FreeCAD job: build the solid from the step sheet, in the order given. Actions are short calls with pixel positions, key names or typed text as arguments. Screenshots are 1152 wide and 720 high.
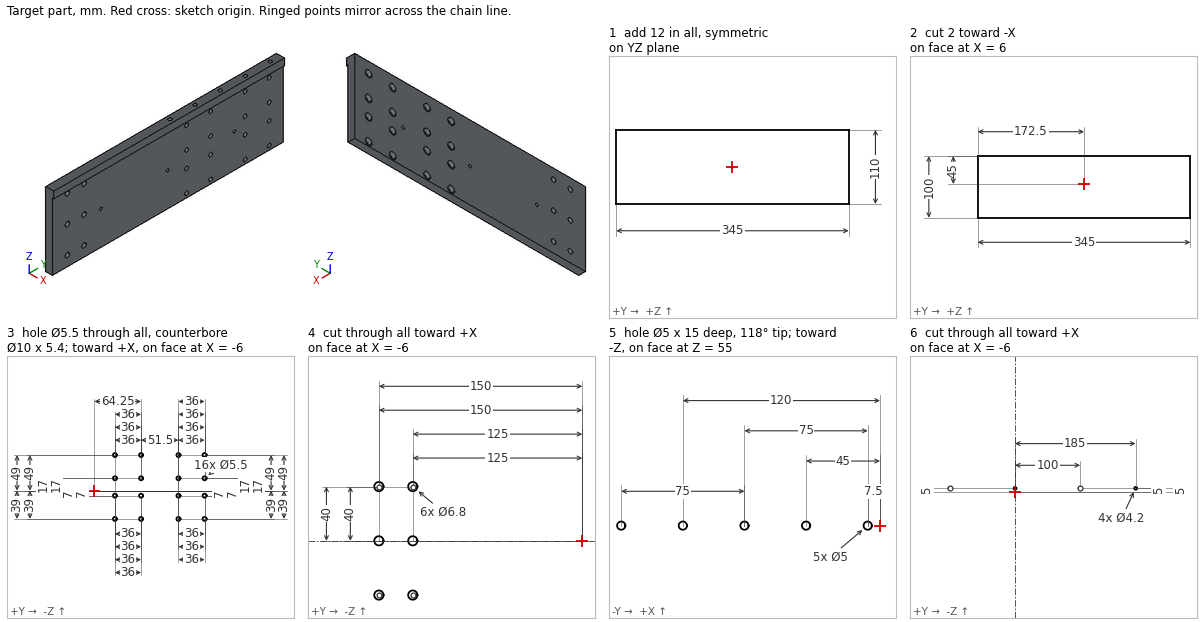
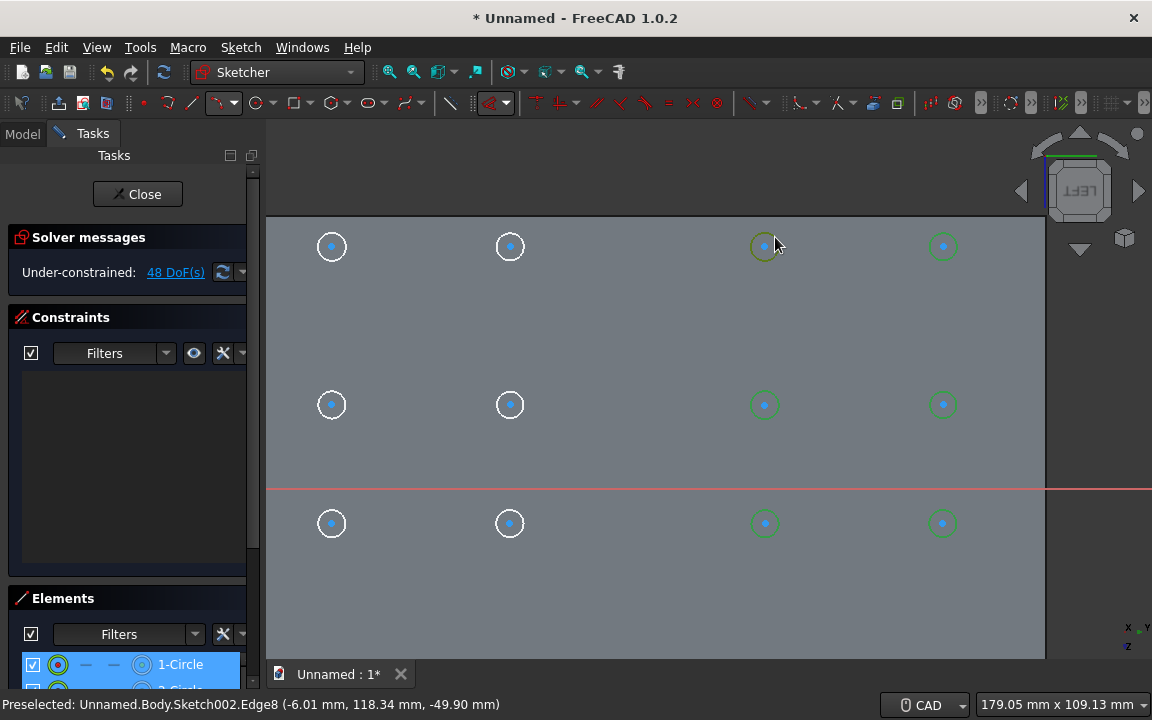
click(520, 237)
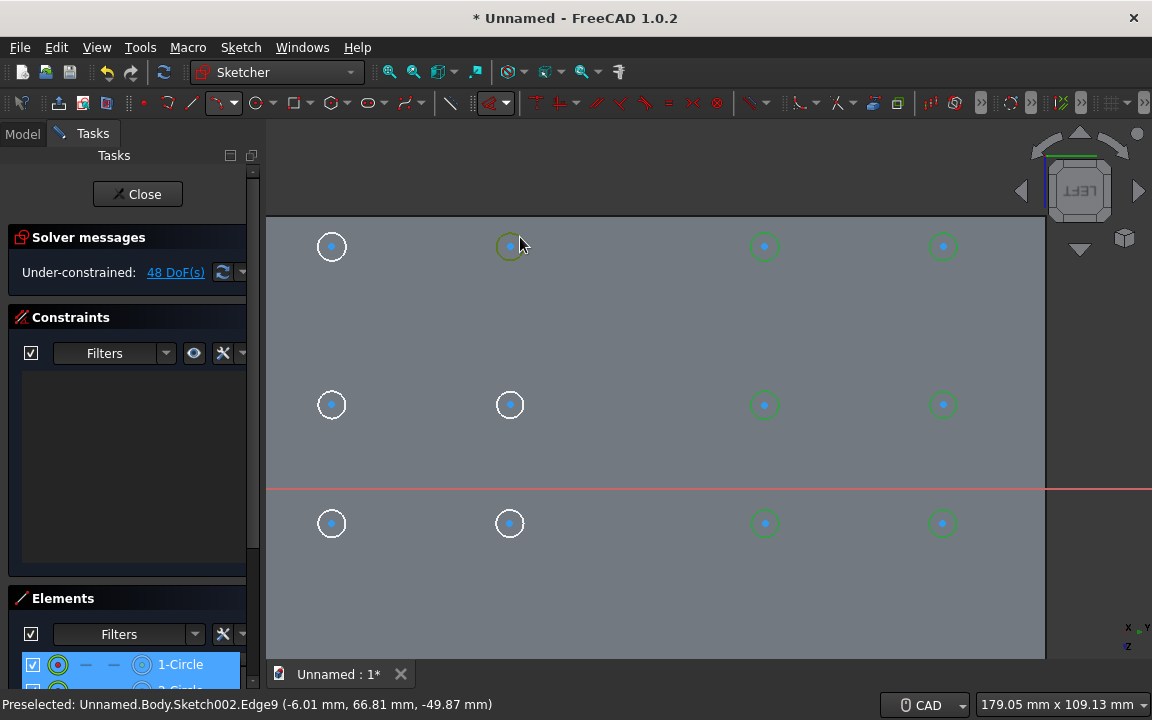
click(342, 237)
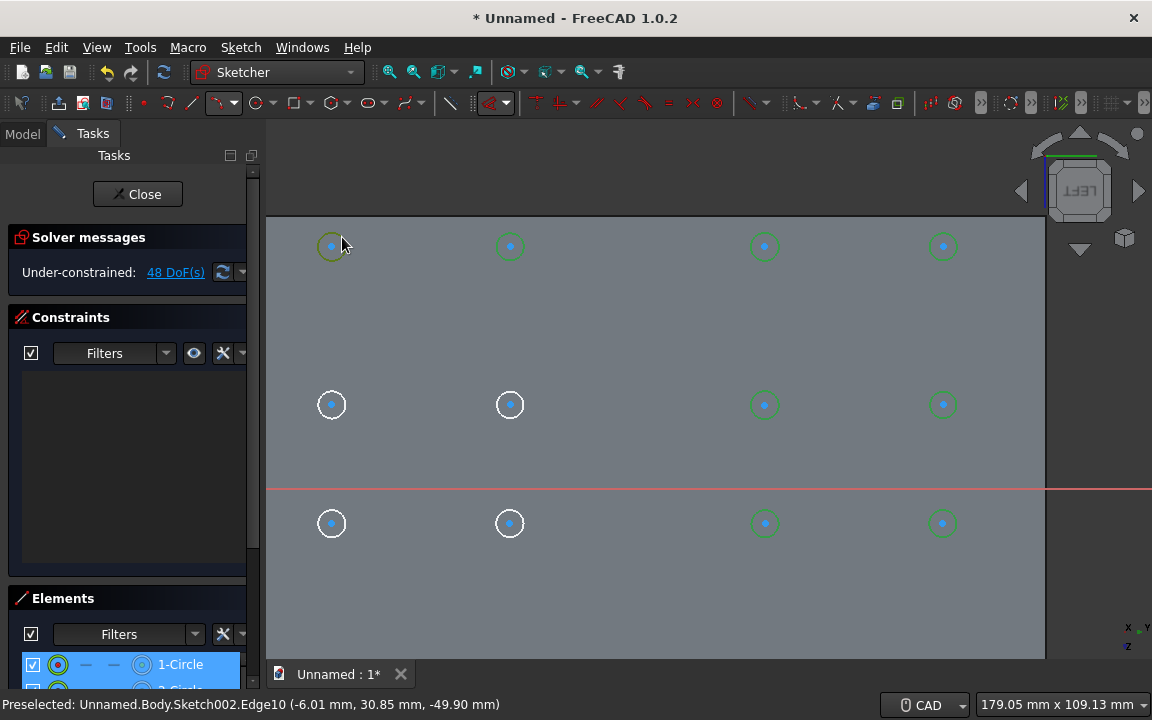
click(520, 396)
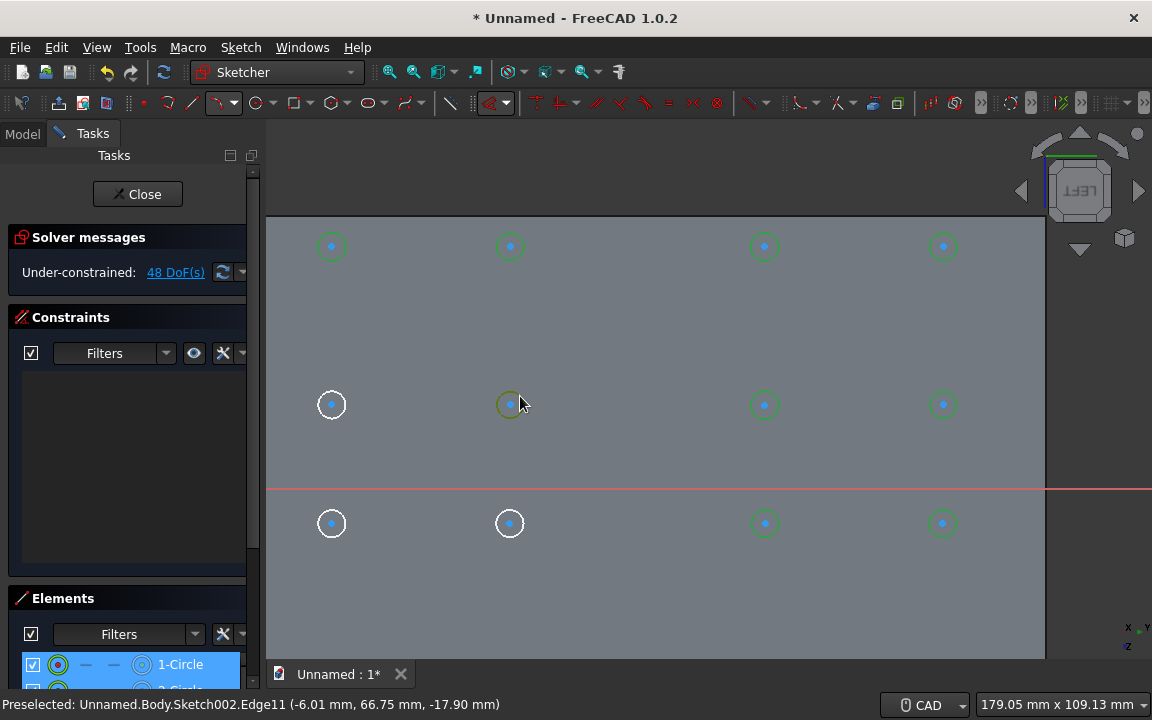
click(341, 395)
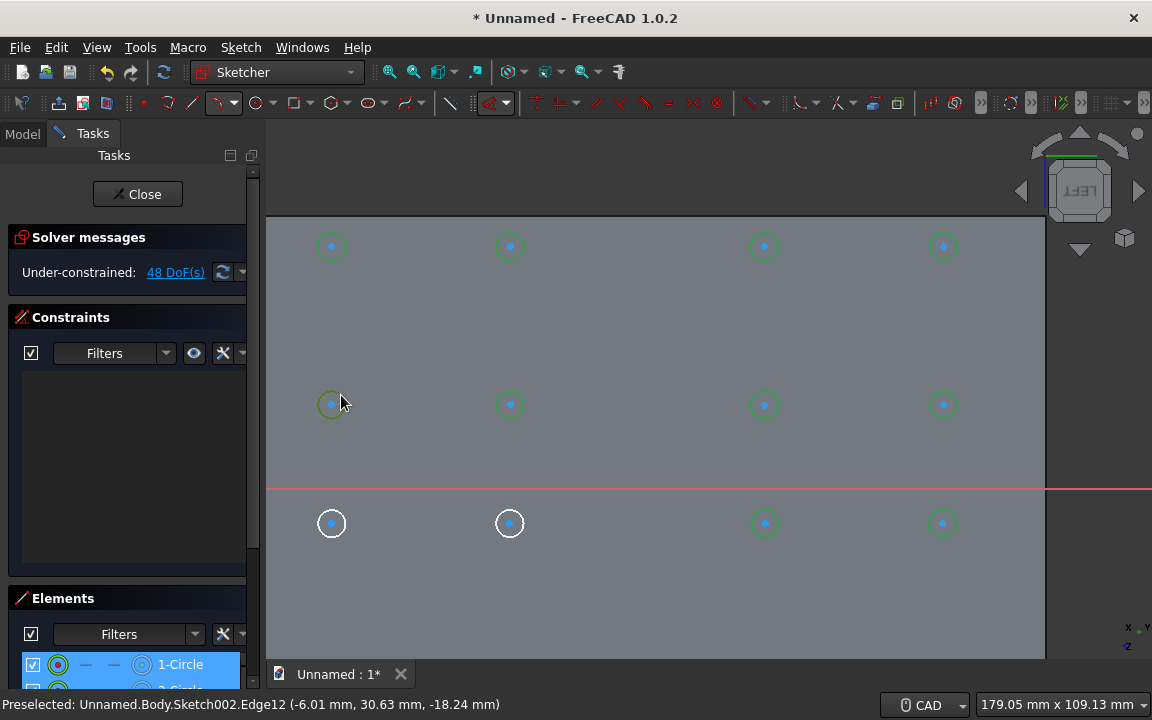
click(519, 514)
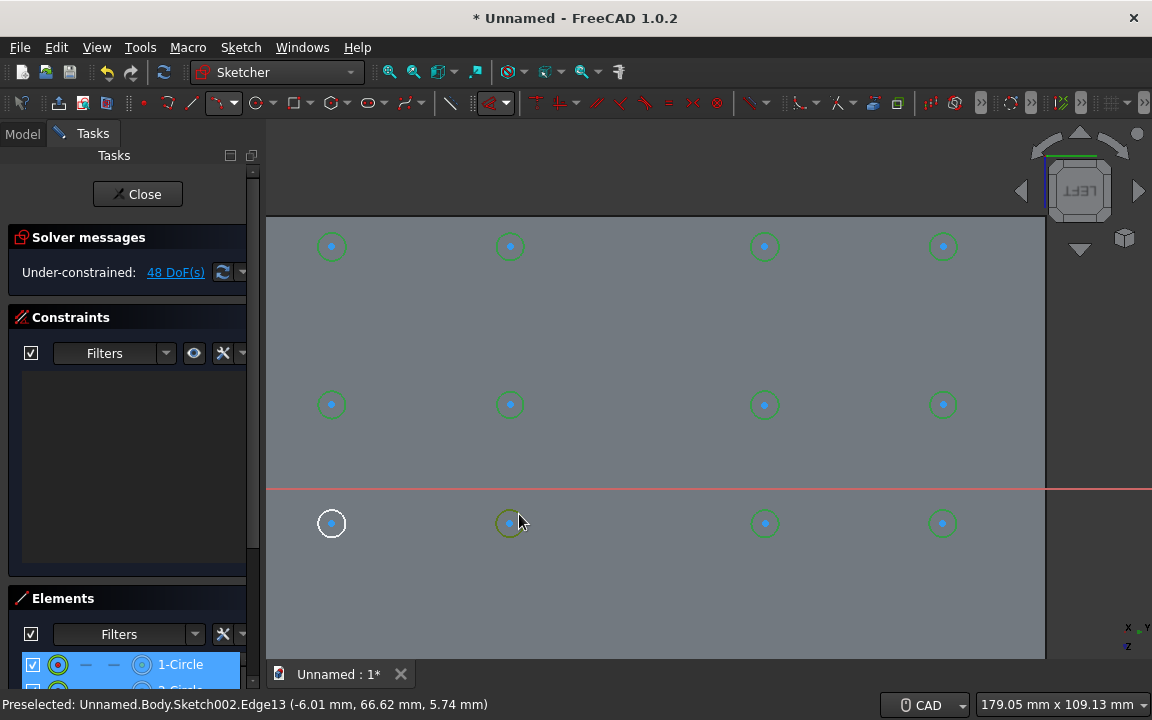
click(341, 514)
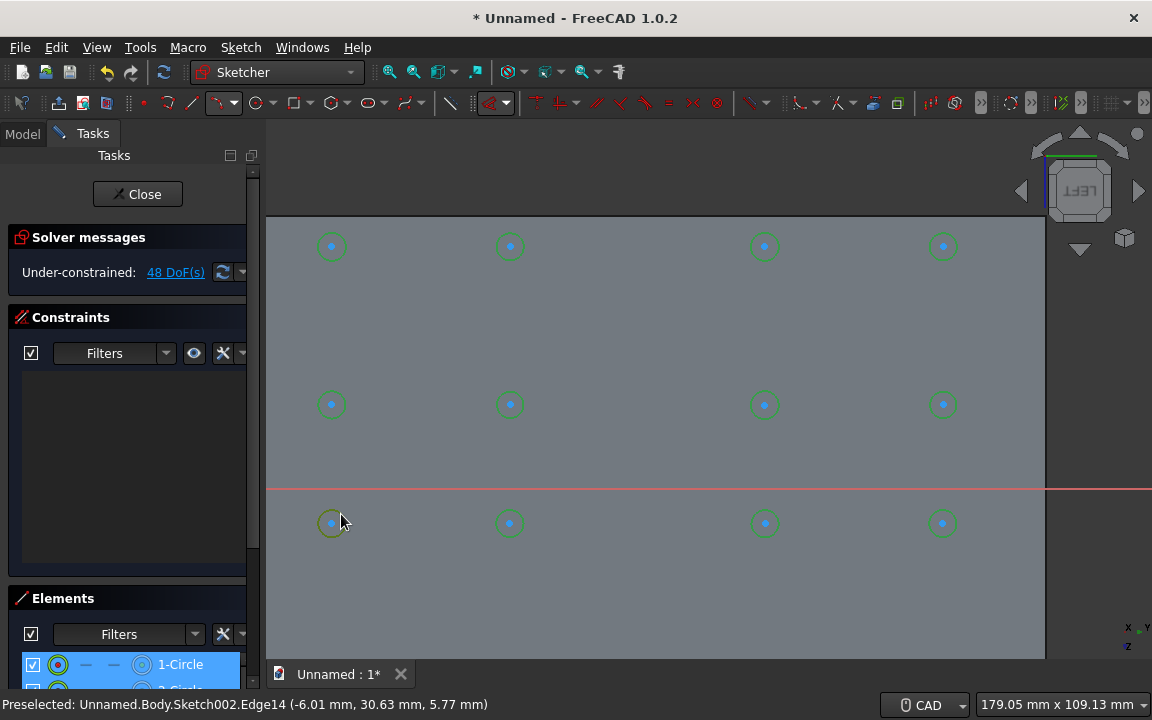
scroll(775, 237, down, 2)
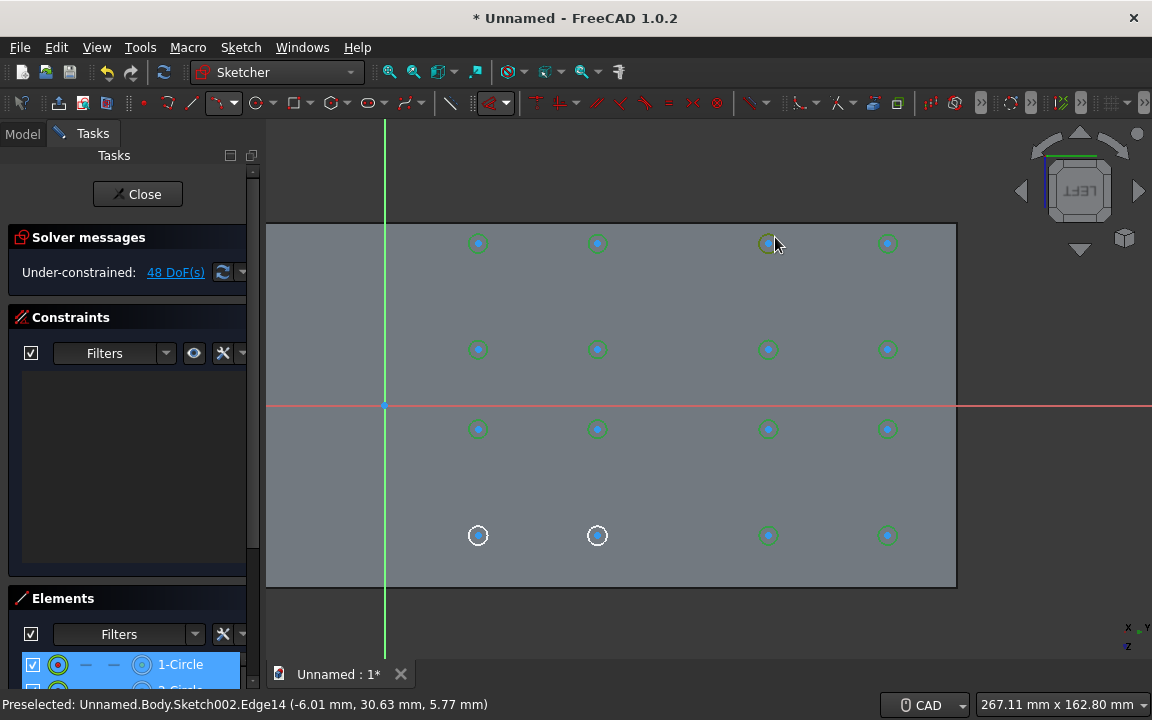
scroll(604, 529, up, 2)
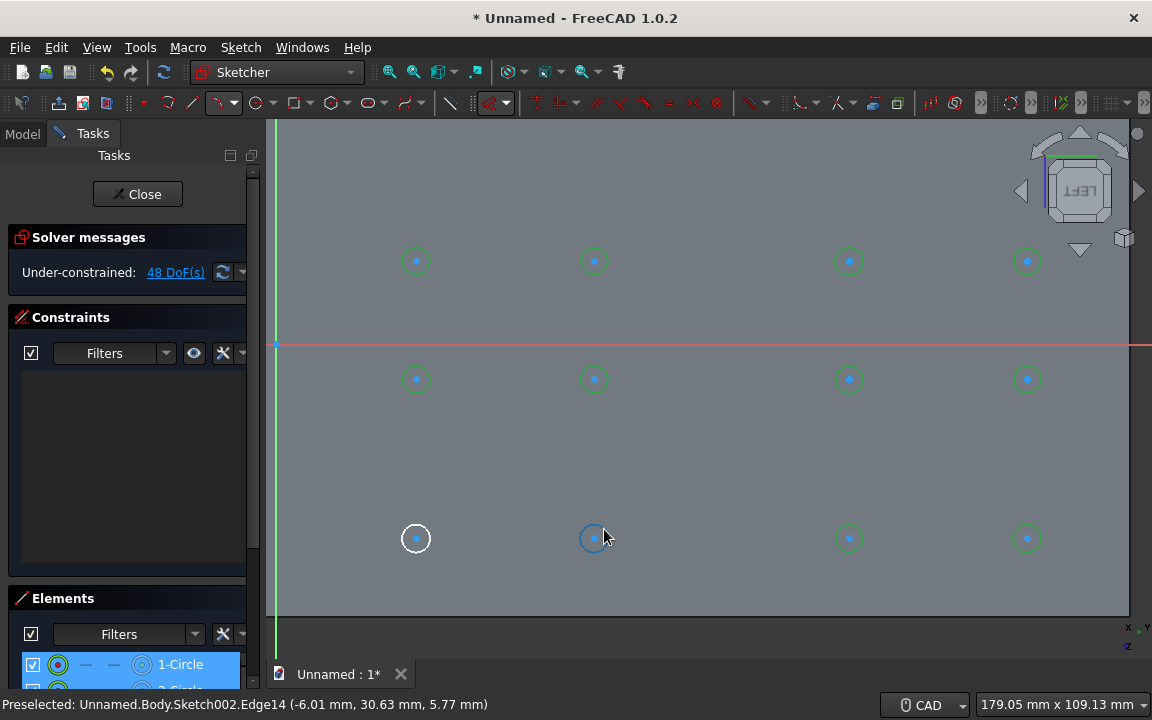
click(604, 529)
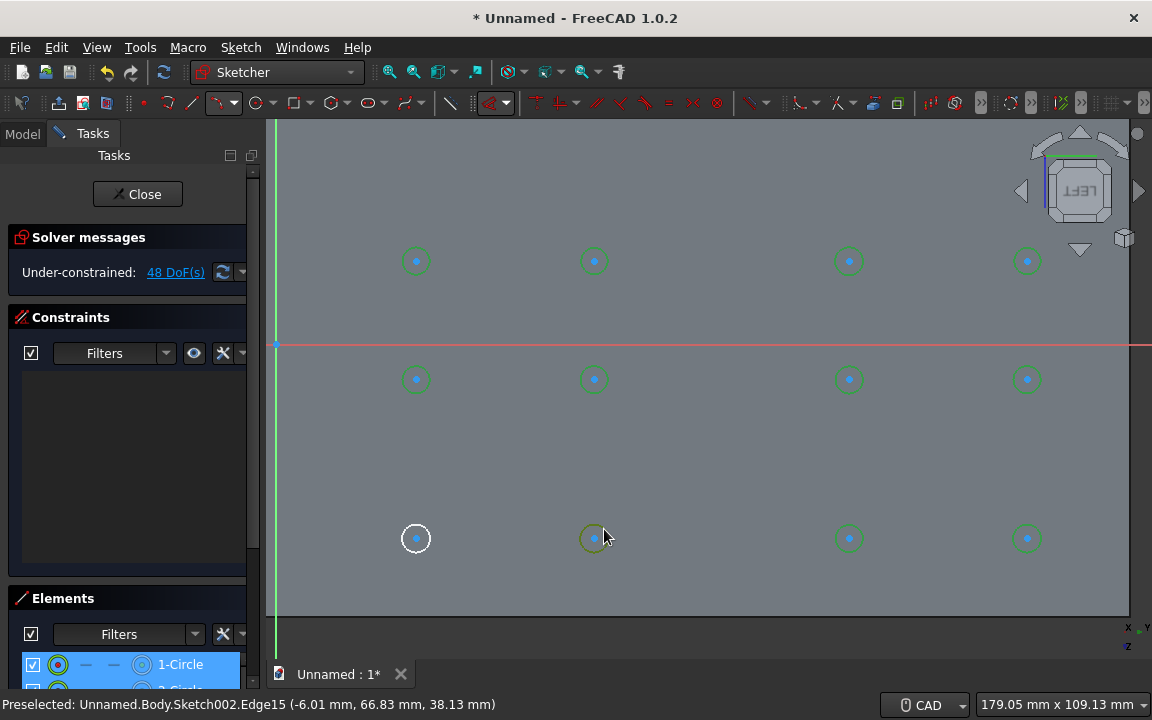
click(426, 529)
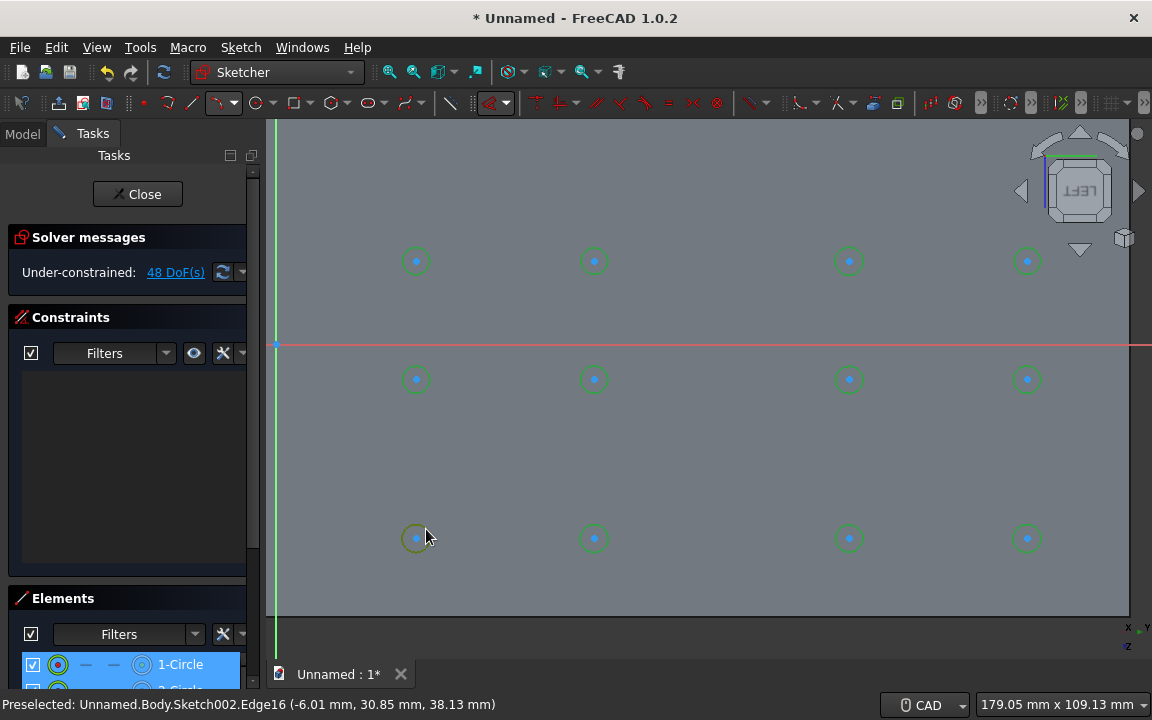
click(670, 104)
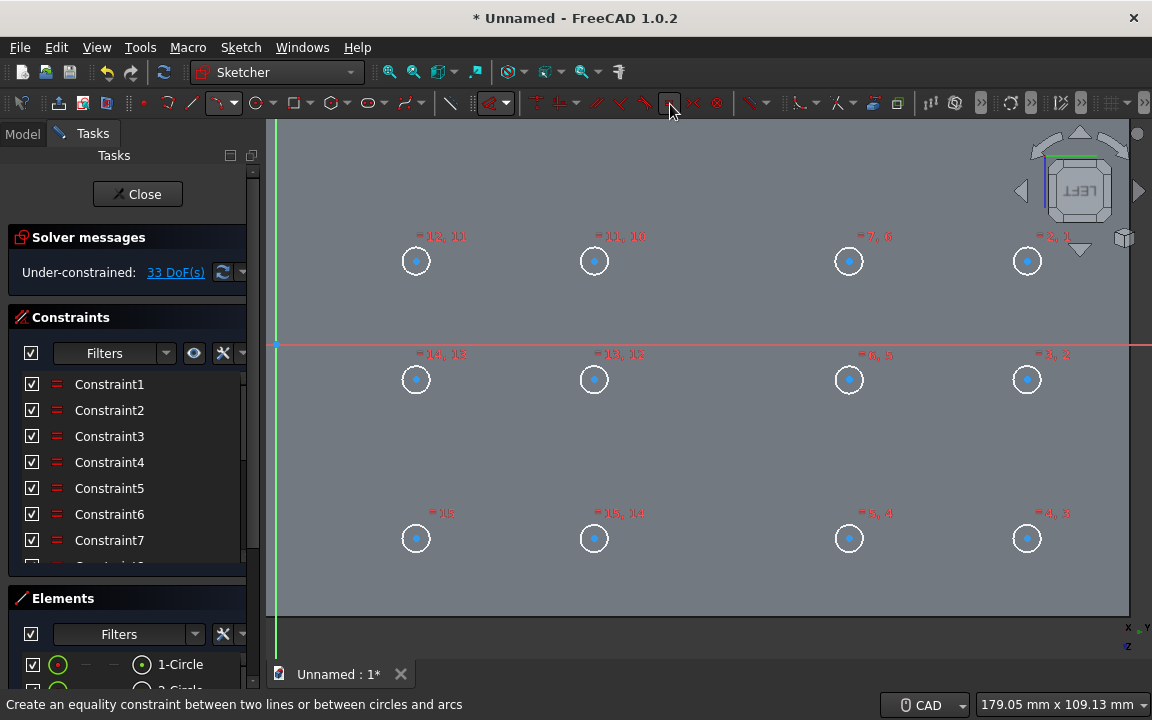
scroll(604, 529, down, 2)